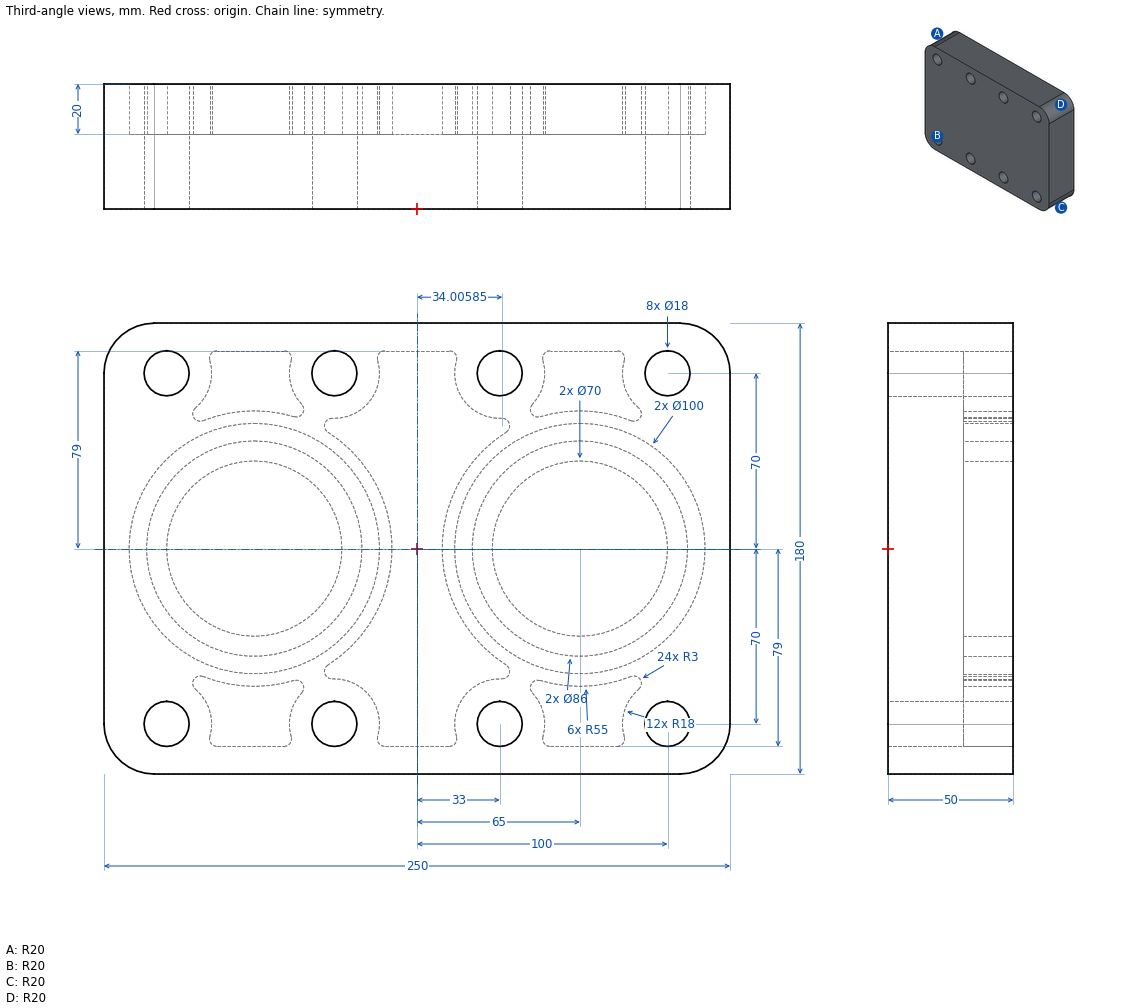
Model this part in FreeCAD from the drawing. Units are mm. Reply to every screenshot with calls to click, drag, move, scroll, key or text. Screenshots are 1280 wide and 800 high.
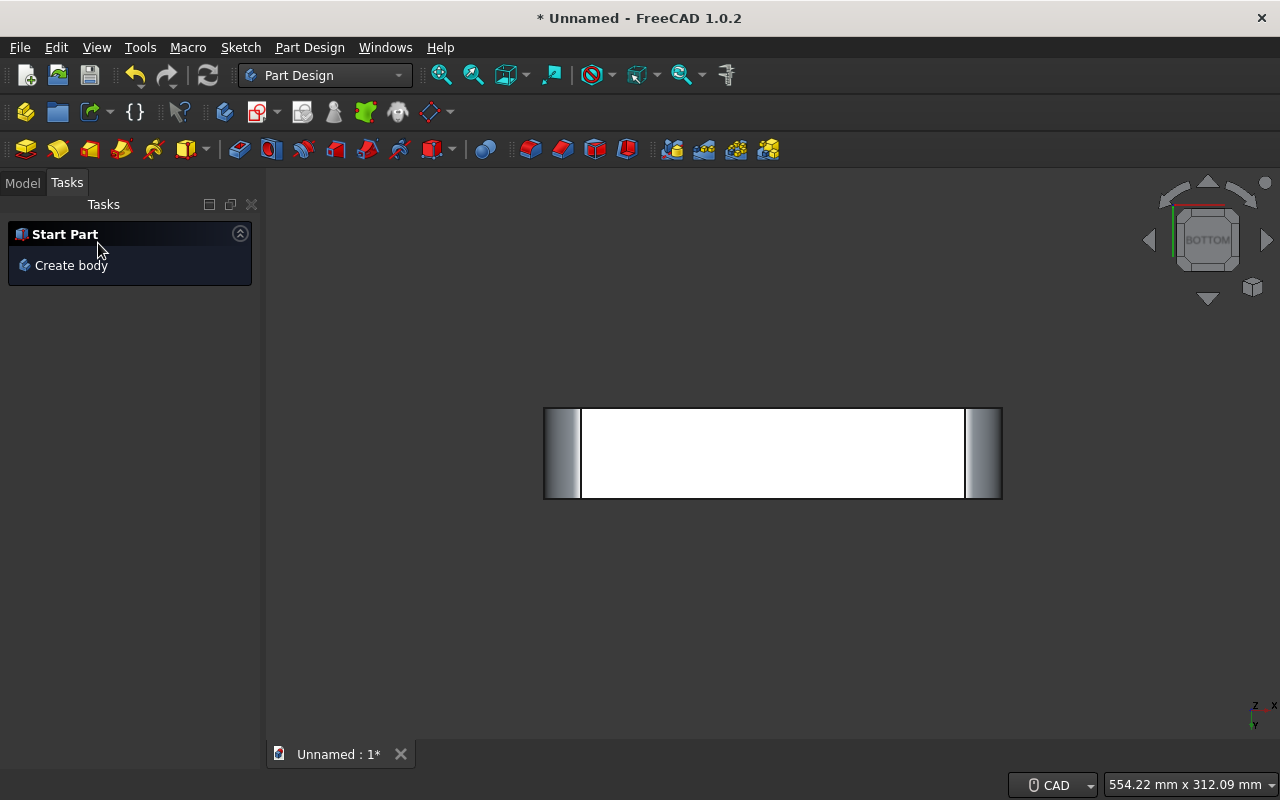
key(0)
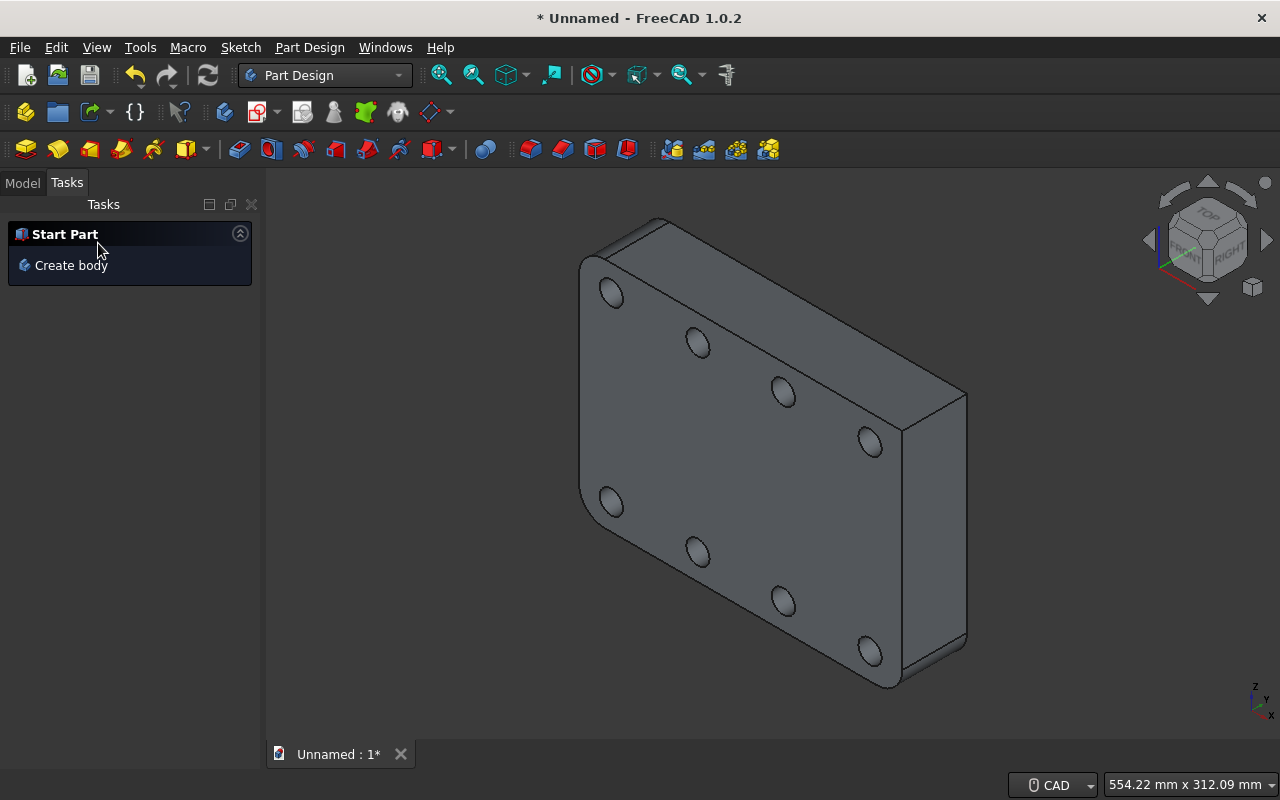
click(935, 411)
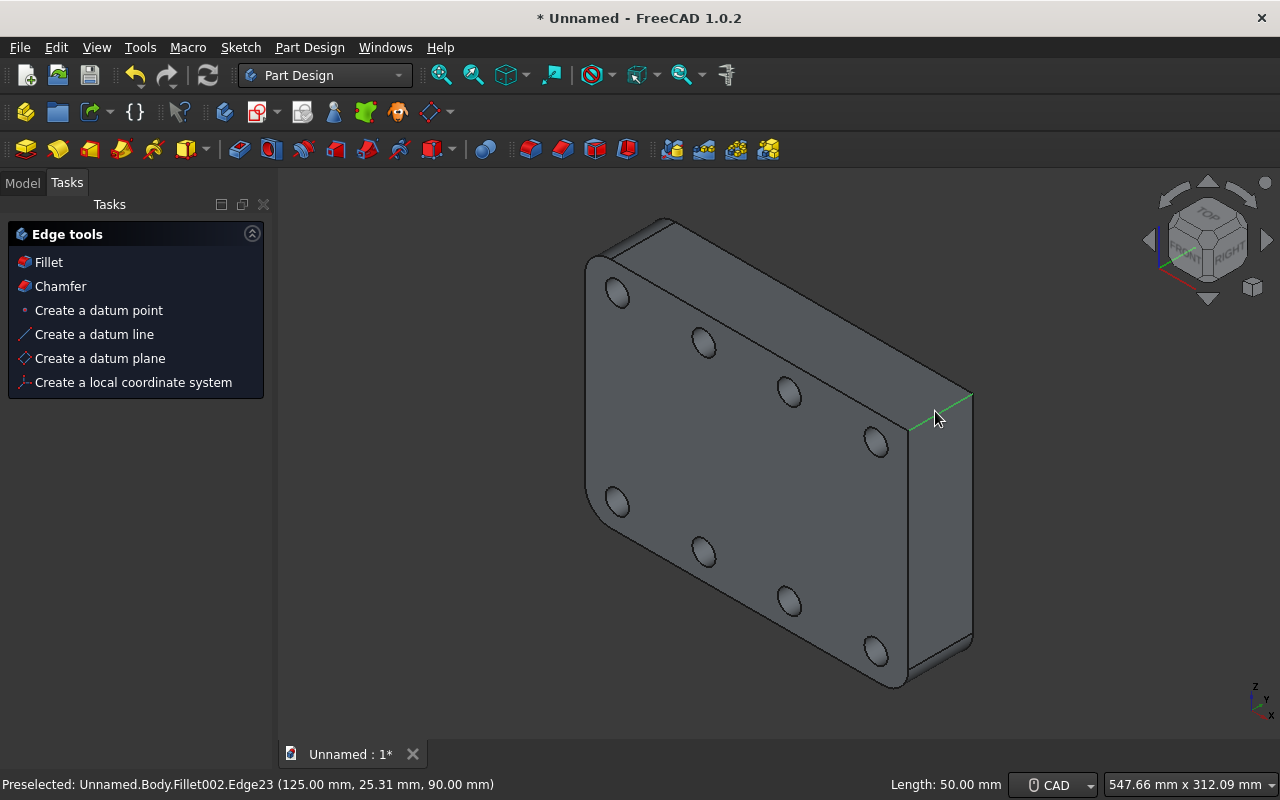
click(532, 150)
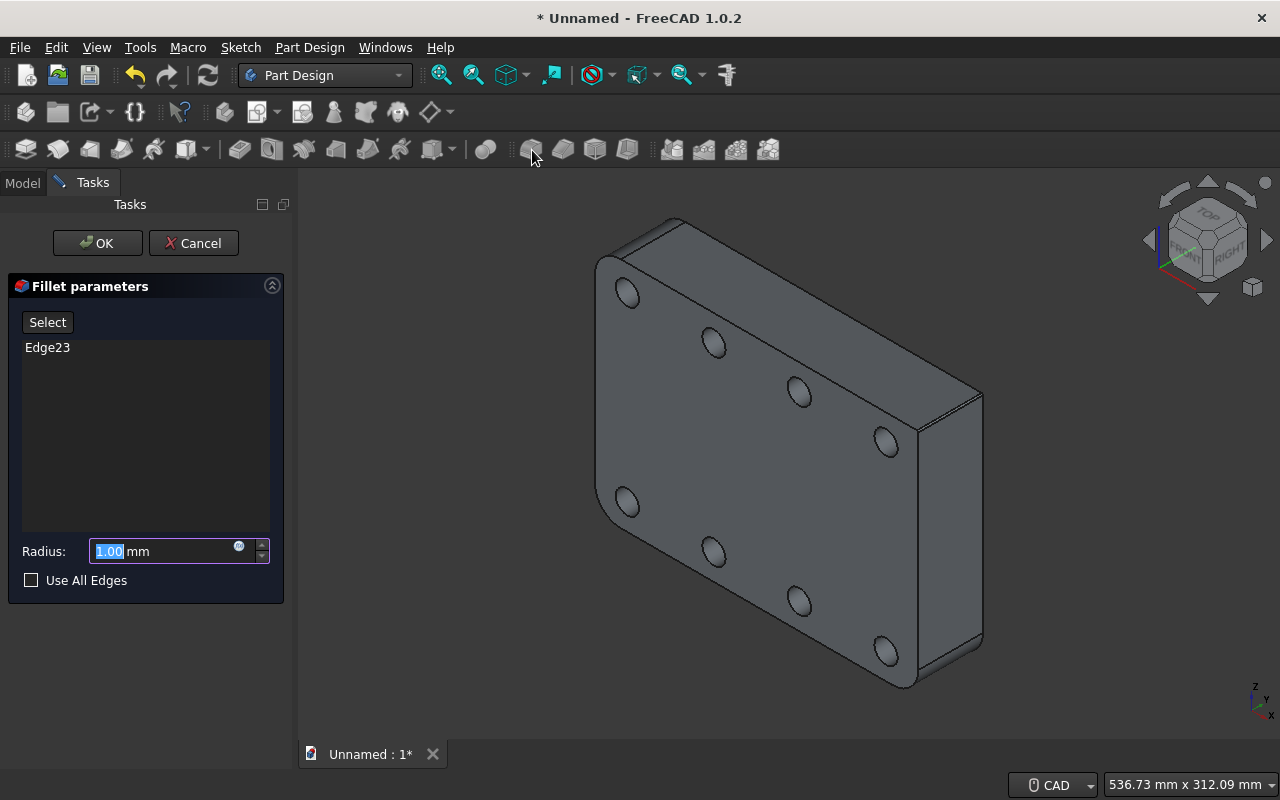
text(20)
key(Tab)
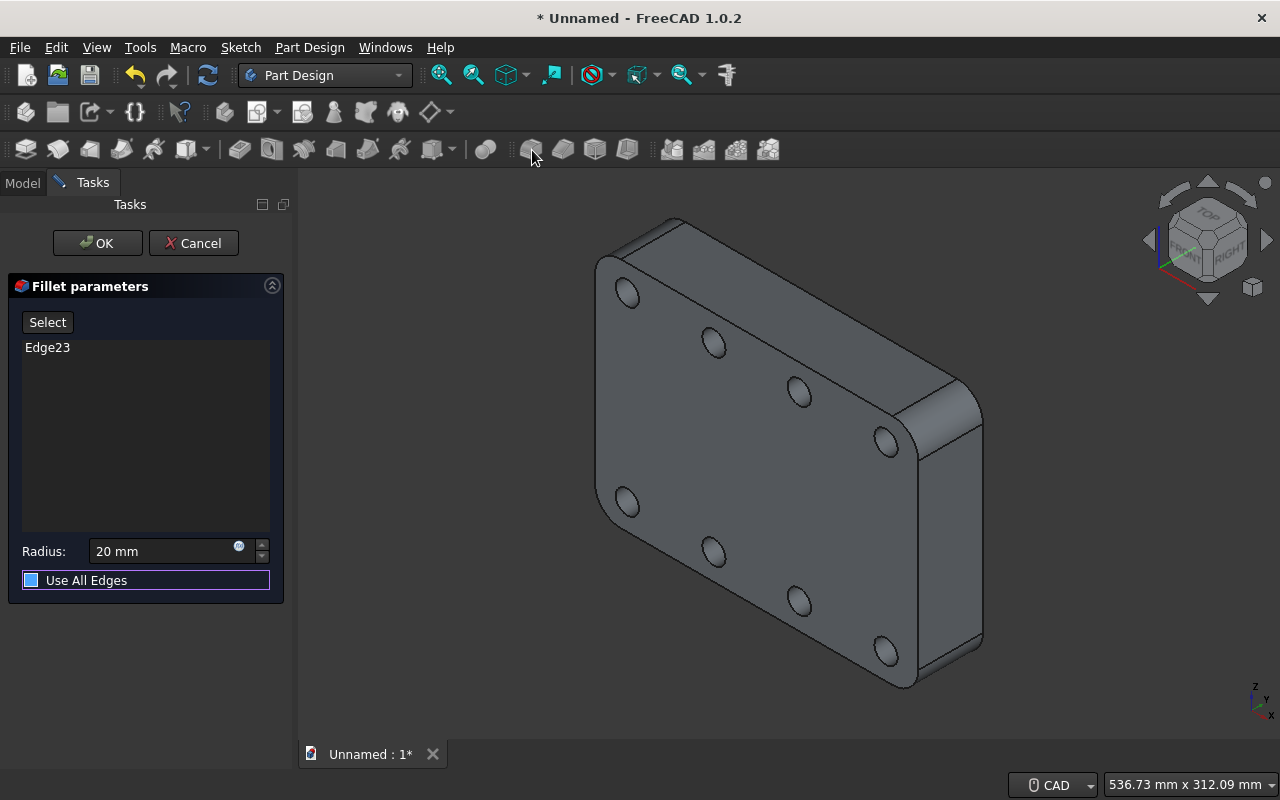
click(98, 243)